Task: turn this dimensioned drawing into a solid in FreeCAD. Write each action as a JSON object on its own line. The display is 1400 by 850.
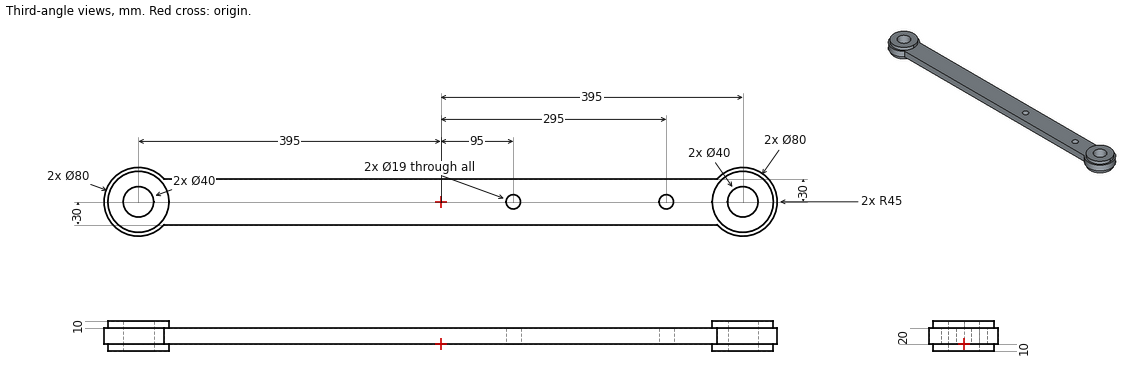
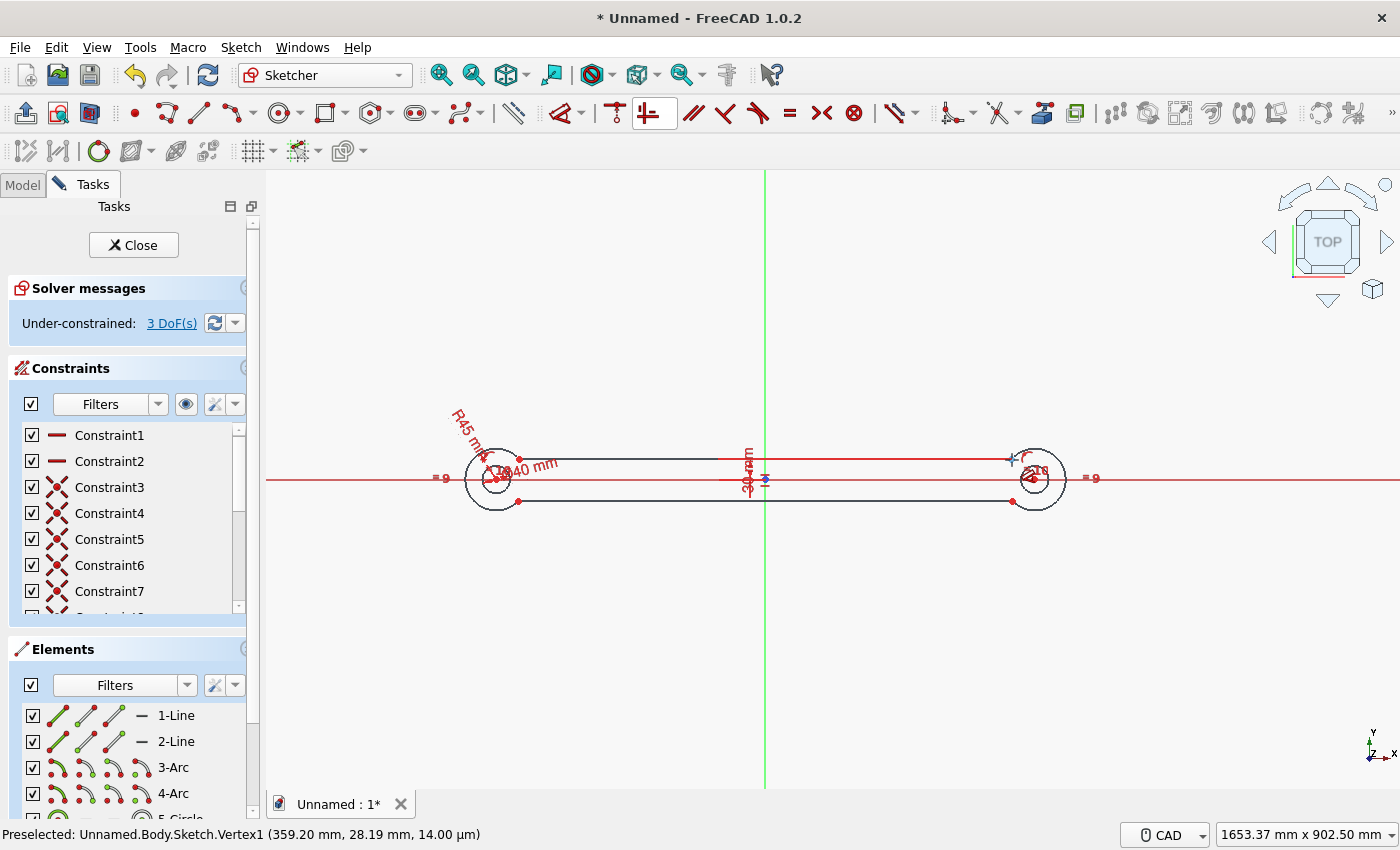
{"action": "scroll", "coordinate": [518, 501], "scroll_direction": "up", "scroll_amount": 4}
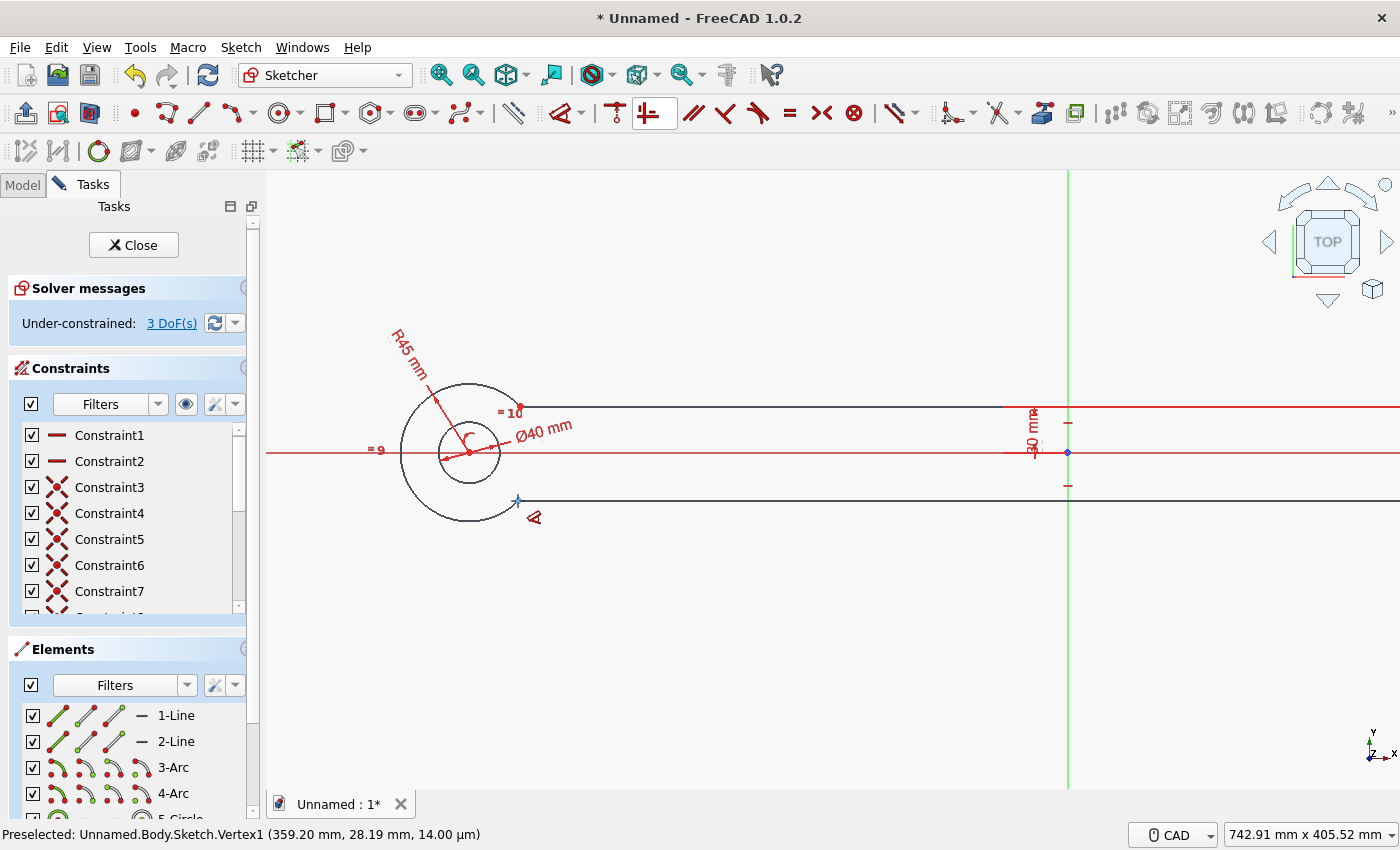
{"action": "left_click", "coordinate": [518, 501]}
{"action": "left_click", "coordinate": [1102, 477]}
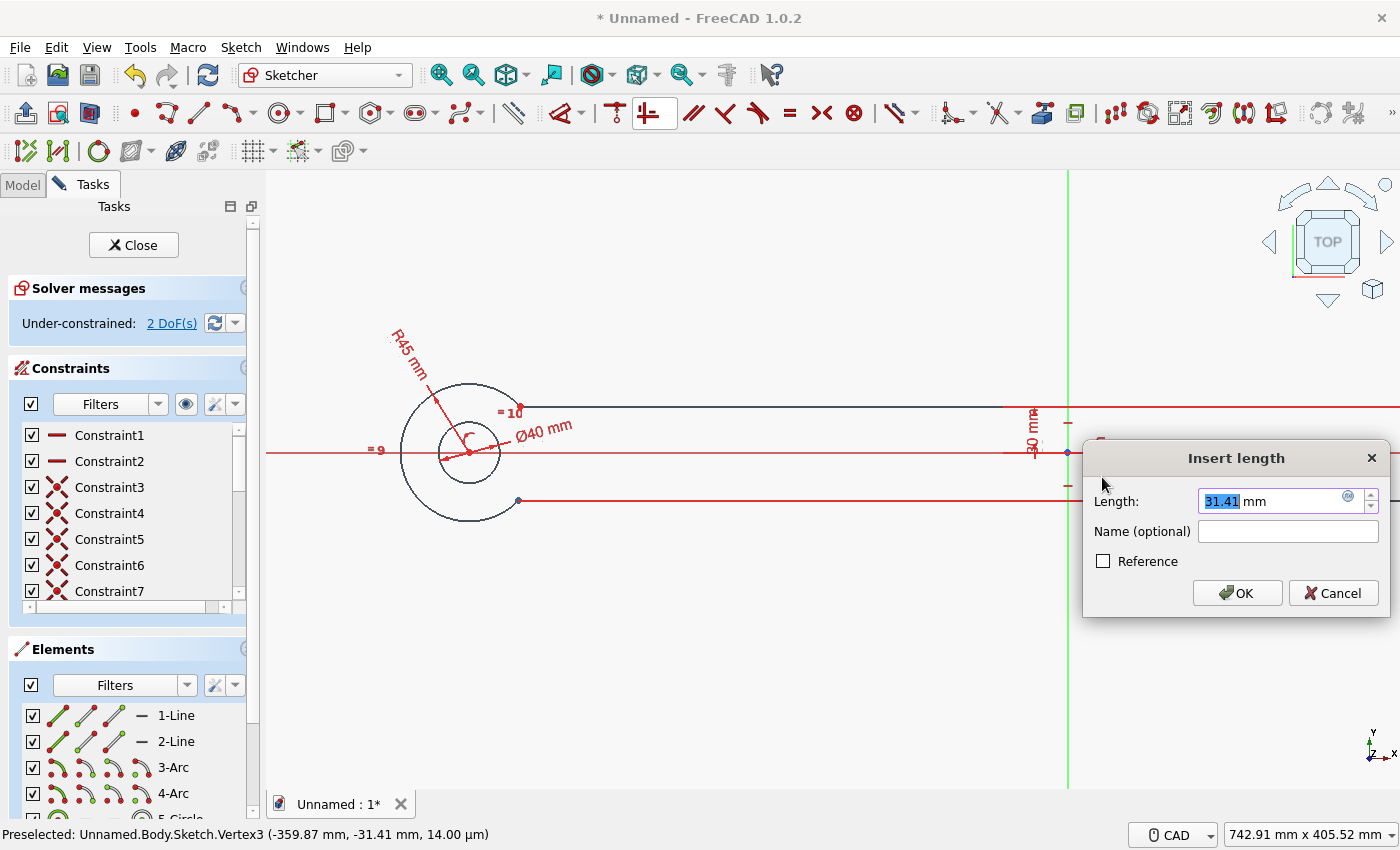
{"action": "type", "text": "30"}
{"action": "key", "text": "Return"}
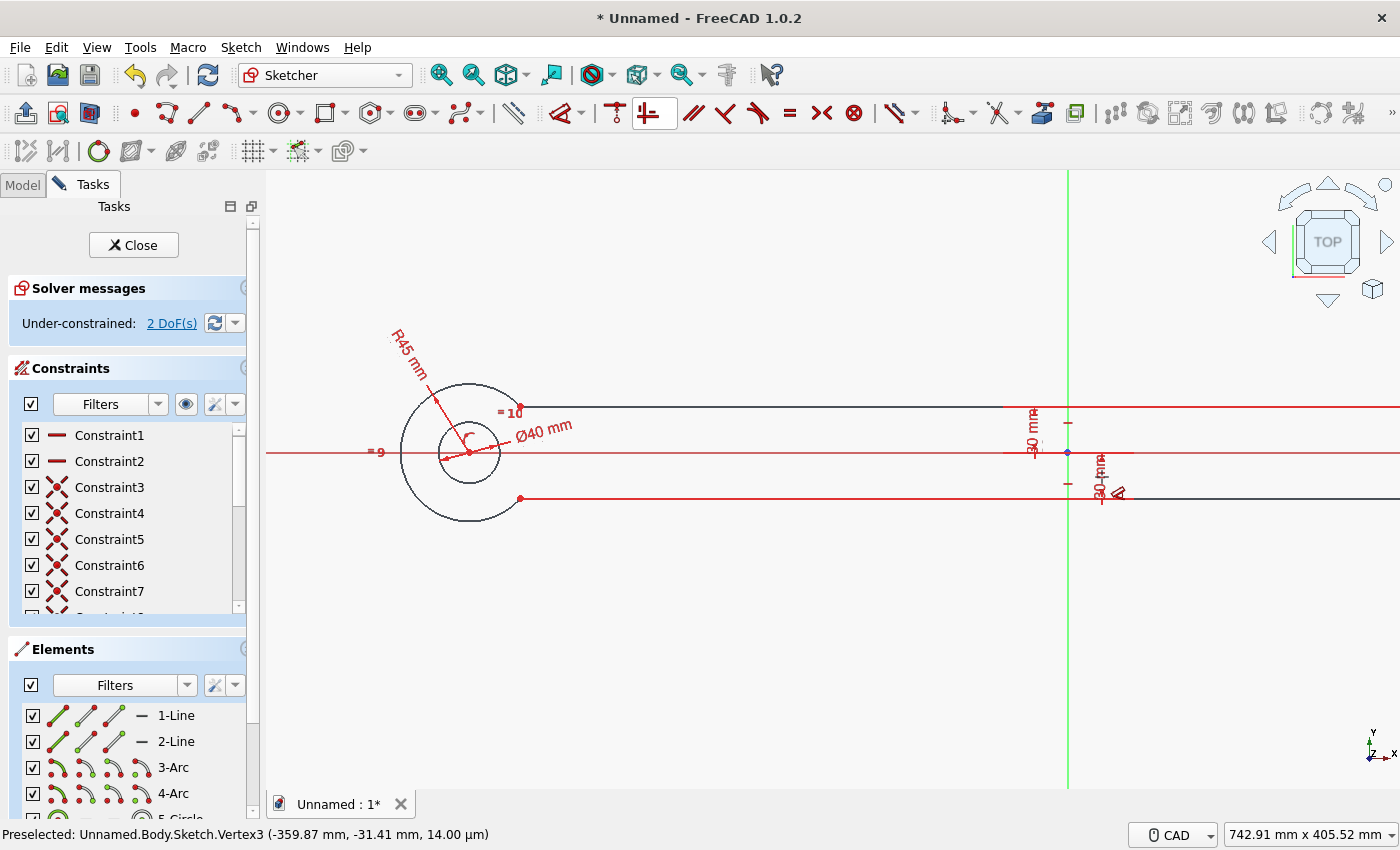
{"action": "left_click", "coordinate": [469, 453]}
{"action": "left_click", "coordinate": [768, 535]}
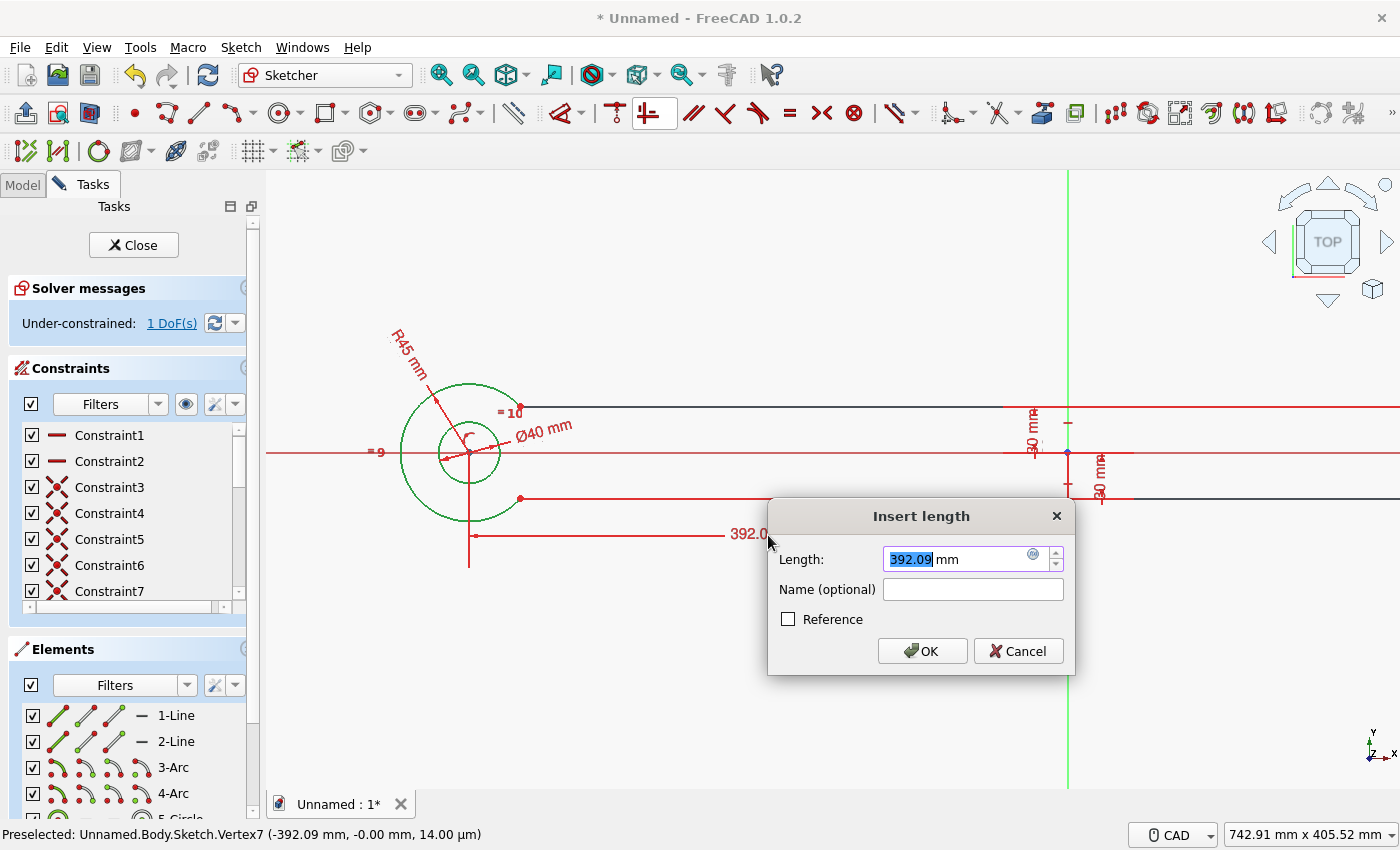
{"action": "type", "text": "395"}
{"action": "key", "text": "Return"}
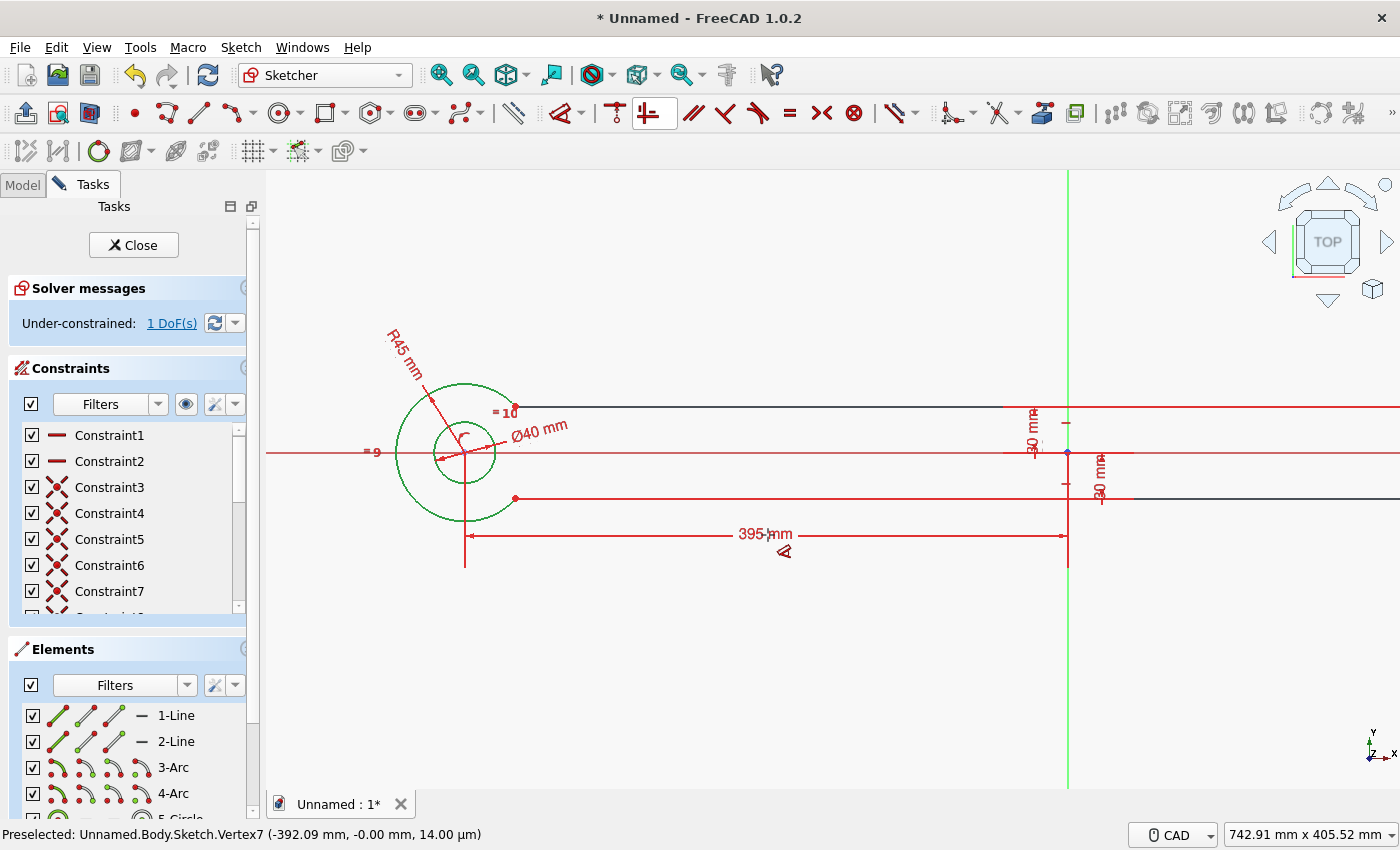
{"action": "scroll", "coordinate": [517, 501], "scroll_direction": "down", "scroll_amount": 4}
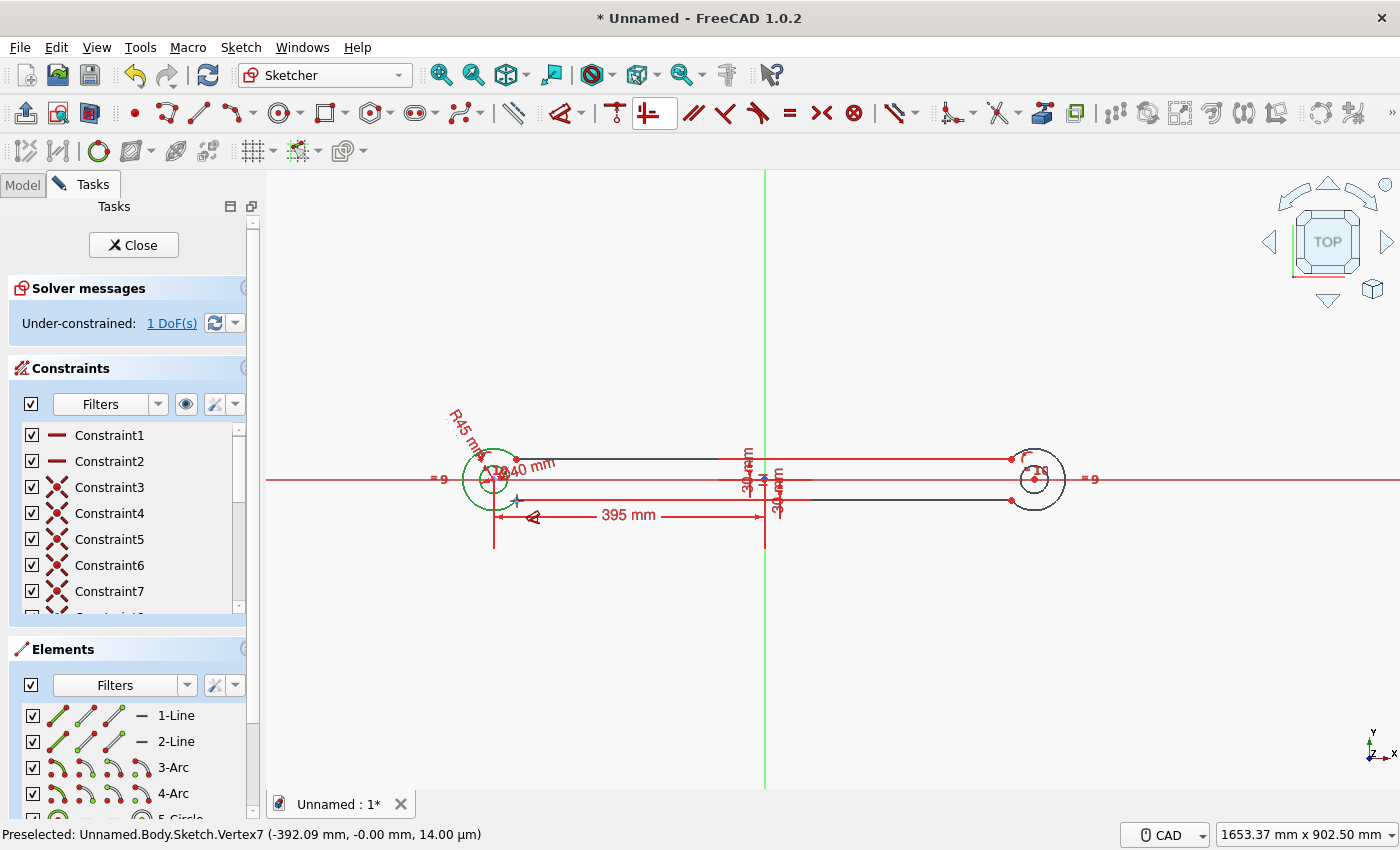
{"action": "left_click", "coordinate": [1034, 480]}
{"action": "left_click", "coordinate": [899, 514]}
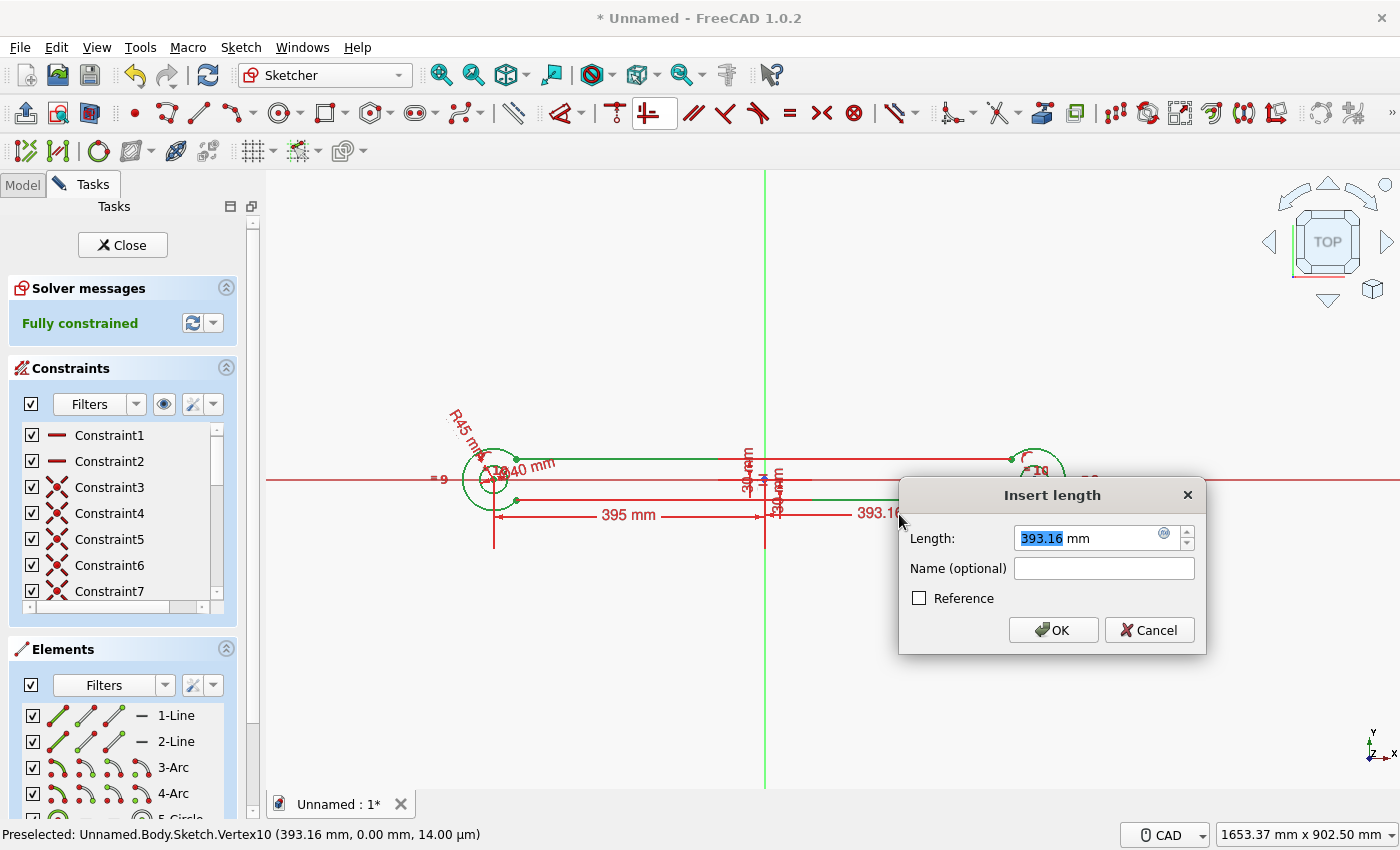
{"action": "type", "text": "395"}
{"action": "key", "text": "Return"}
{"action": "key", "text": "Escape"}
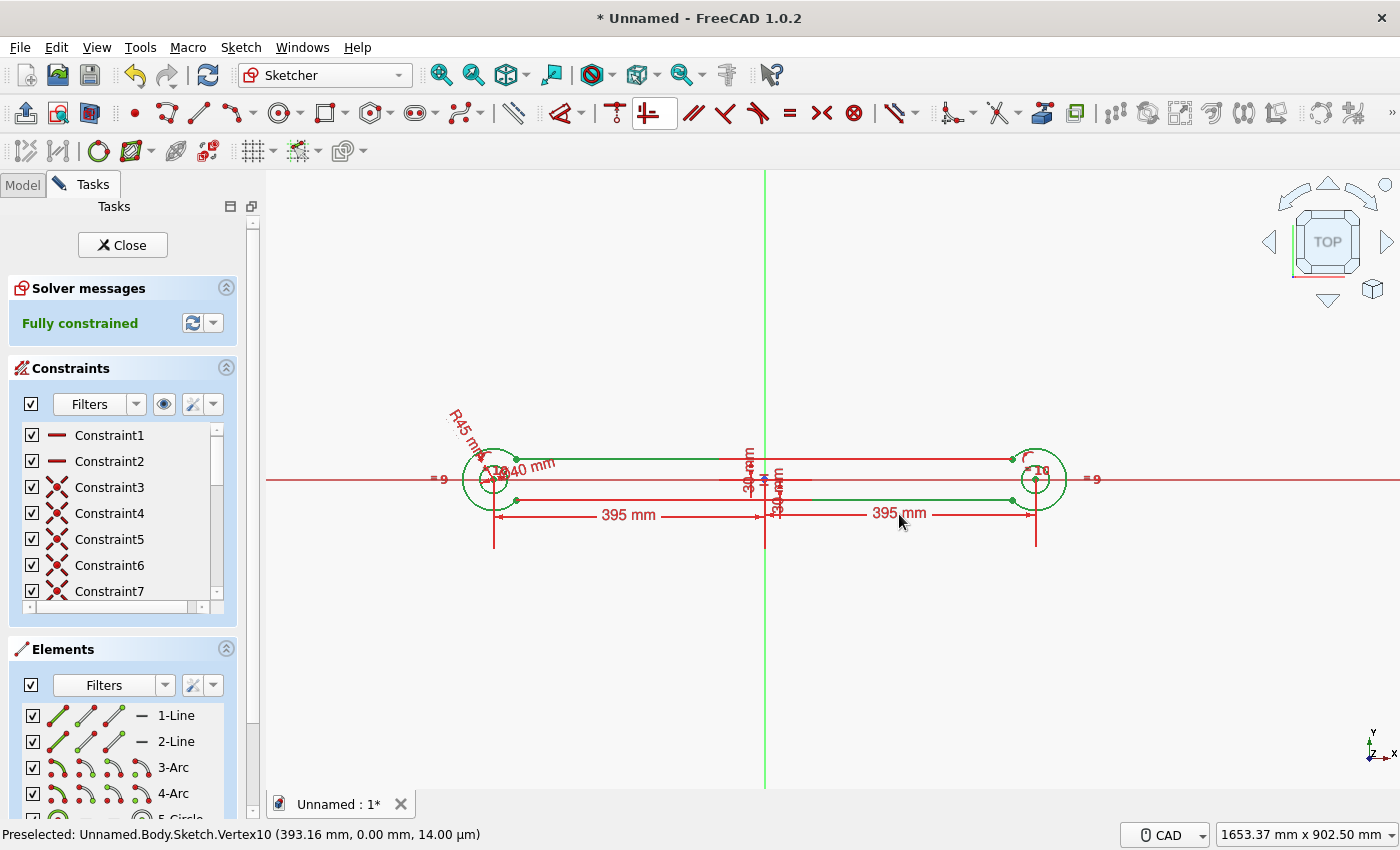
{"action": "left_click", "coordinate": [123, 245]}